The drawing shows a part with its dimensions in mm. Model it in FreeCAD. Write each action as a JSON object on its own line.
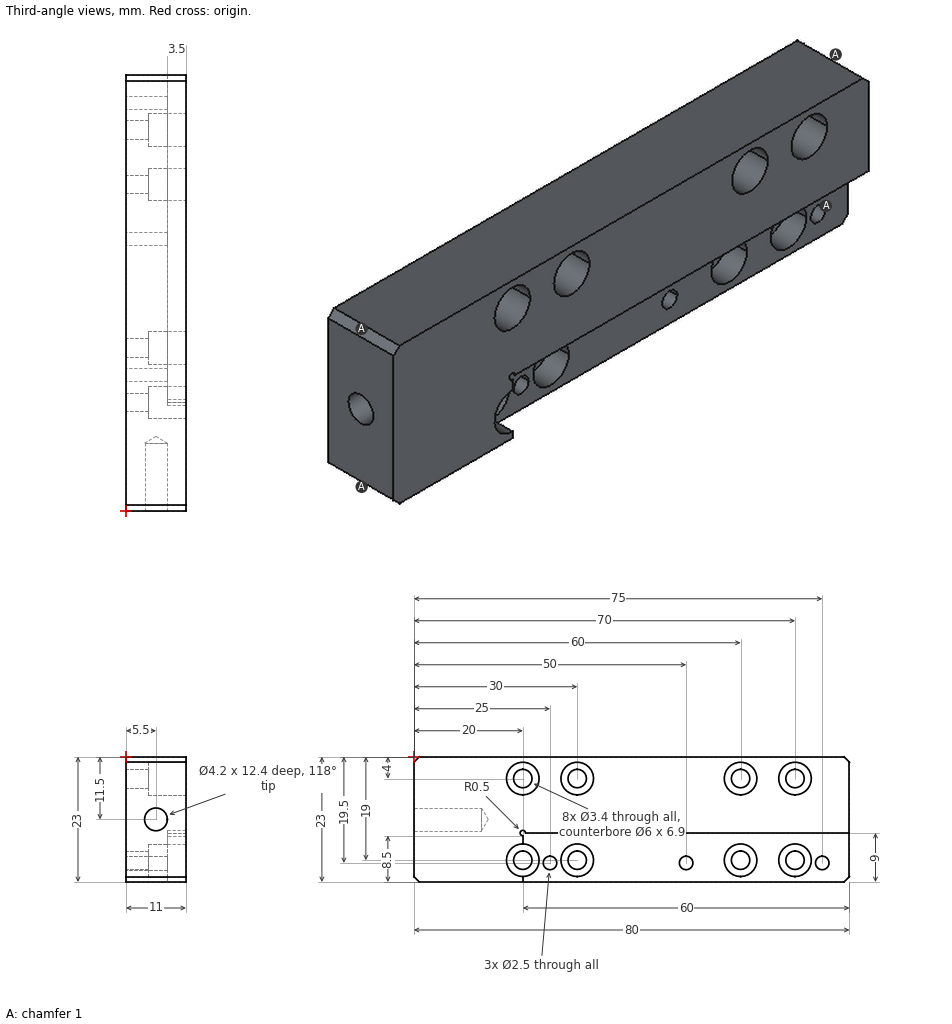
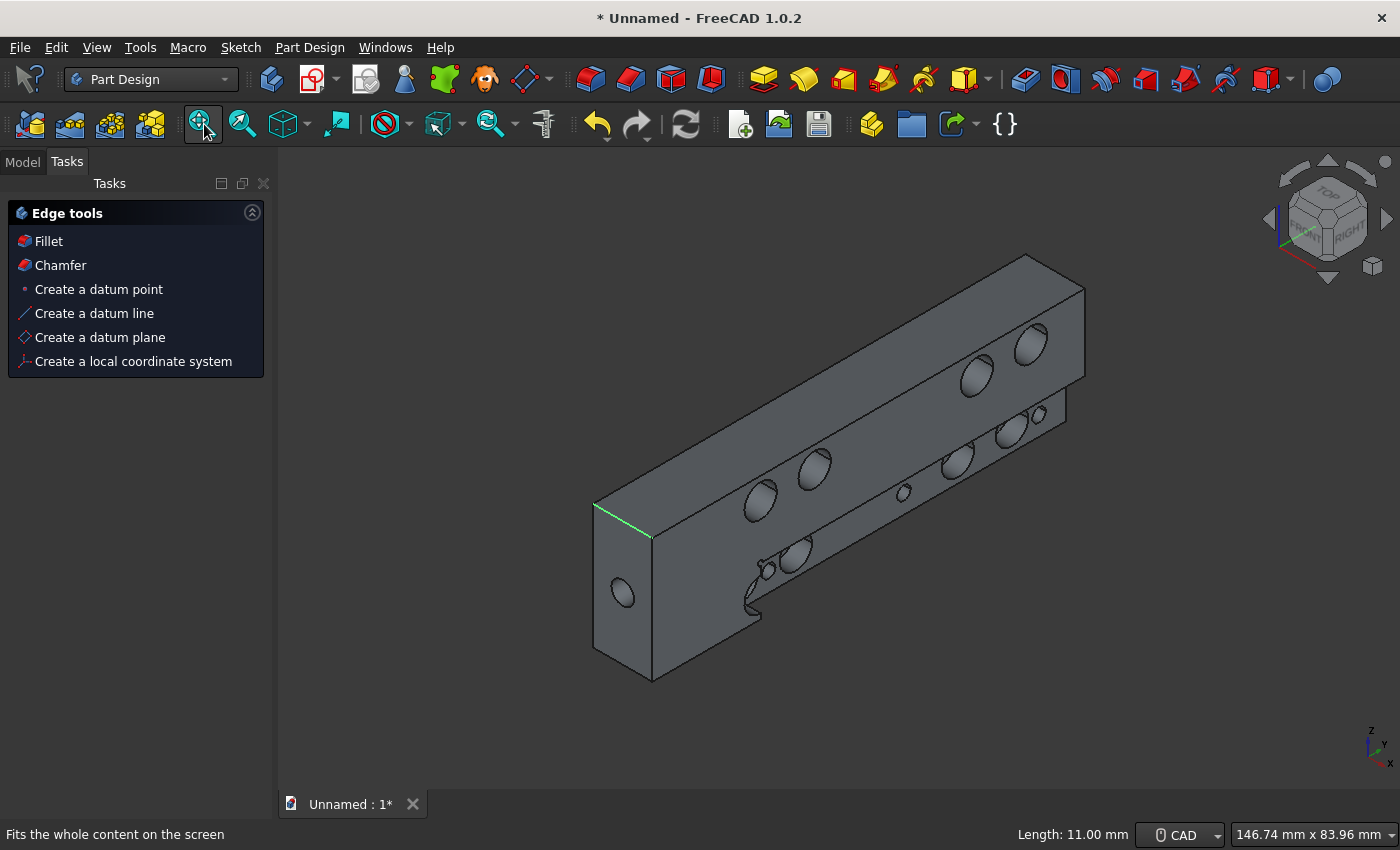
{"action": "key", "text": "1"}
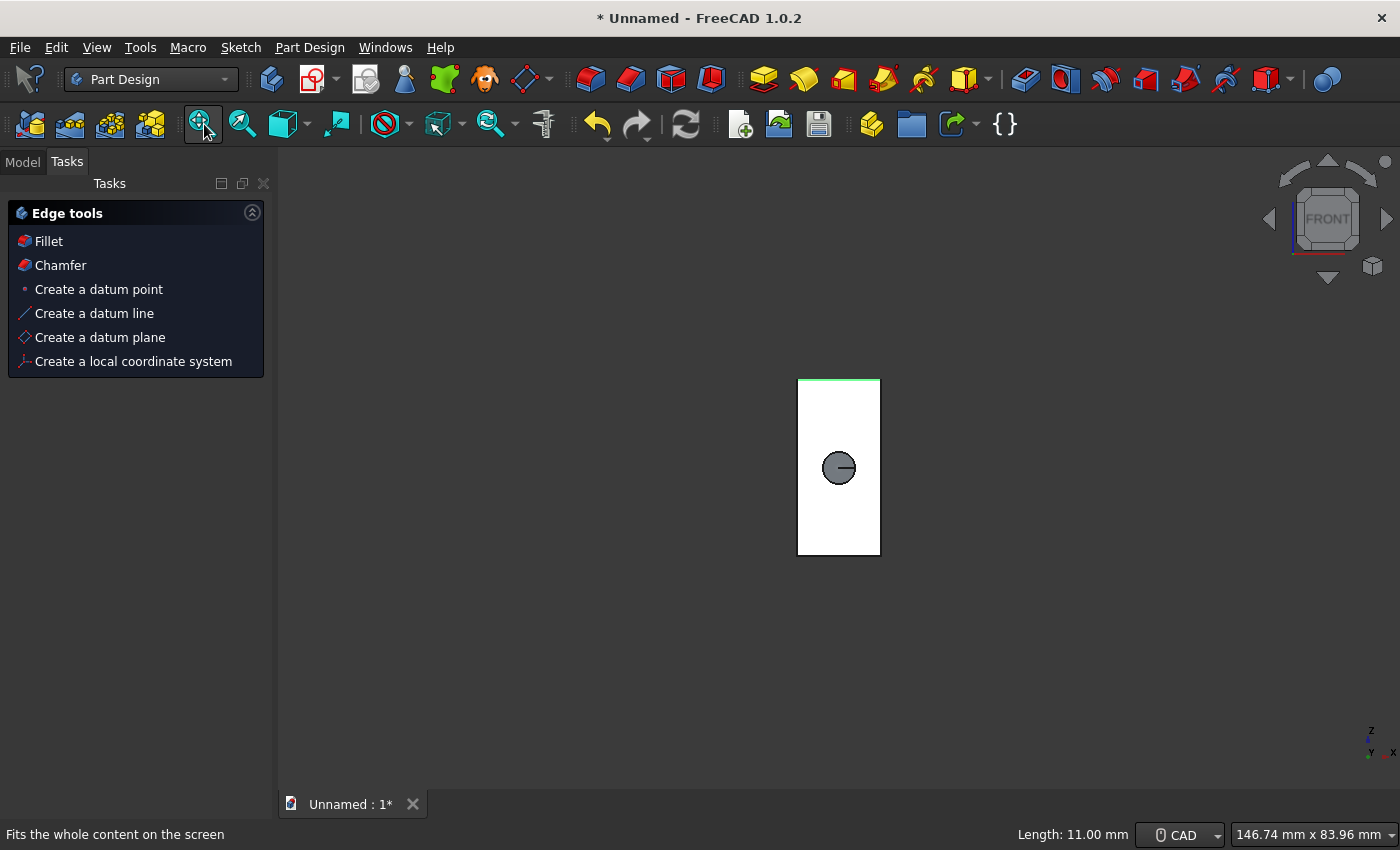
{"action": "left_click", "coordinate": [204, 124]}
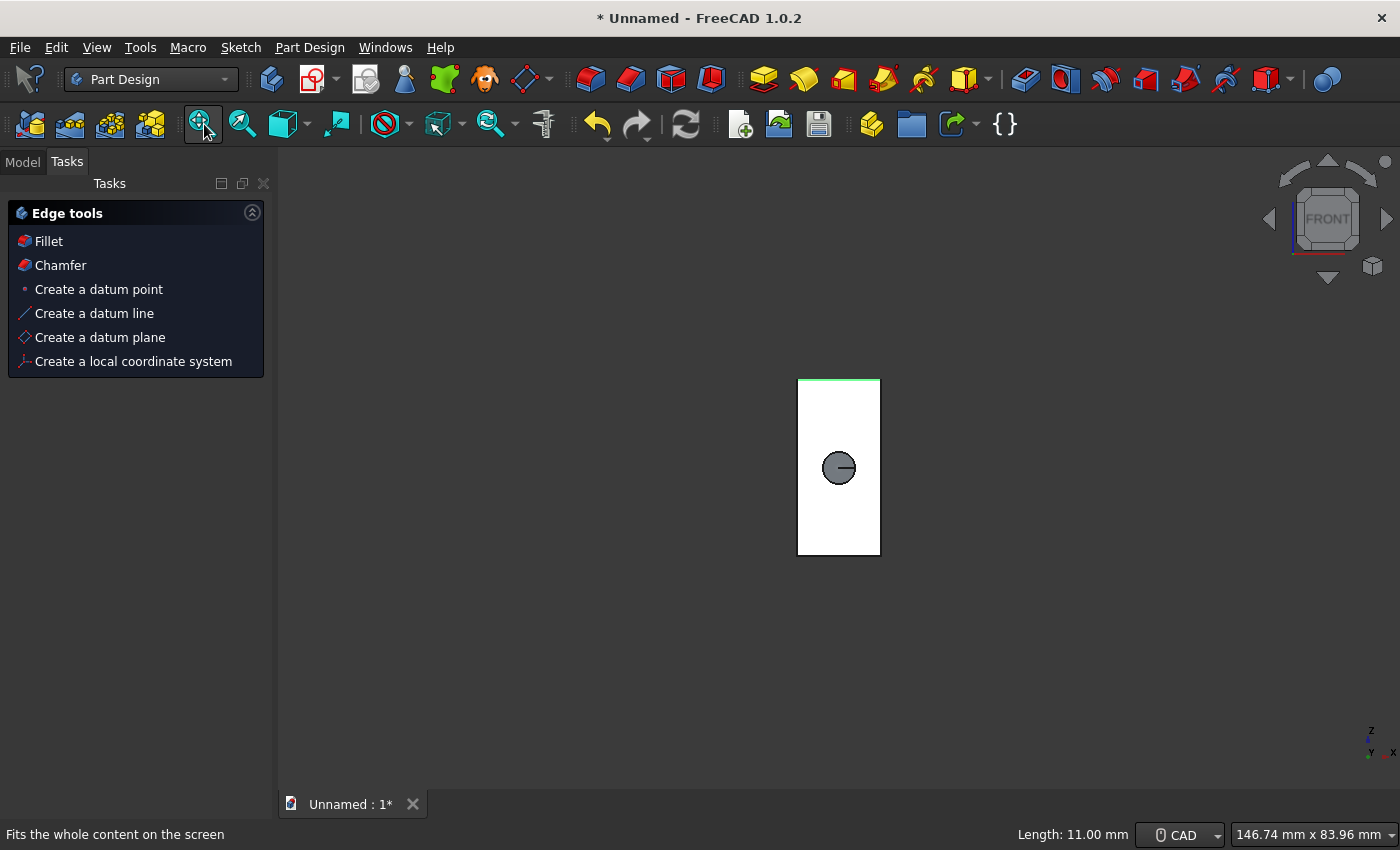
{"action": "key", "text": "3"}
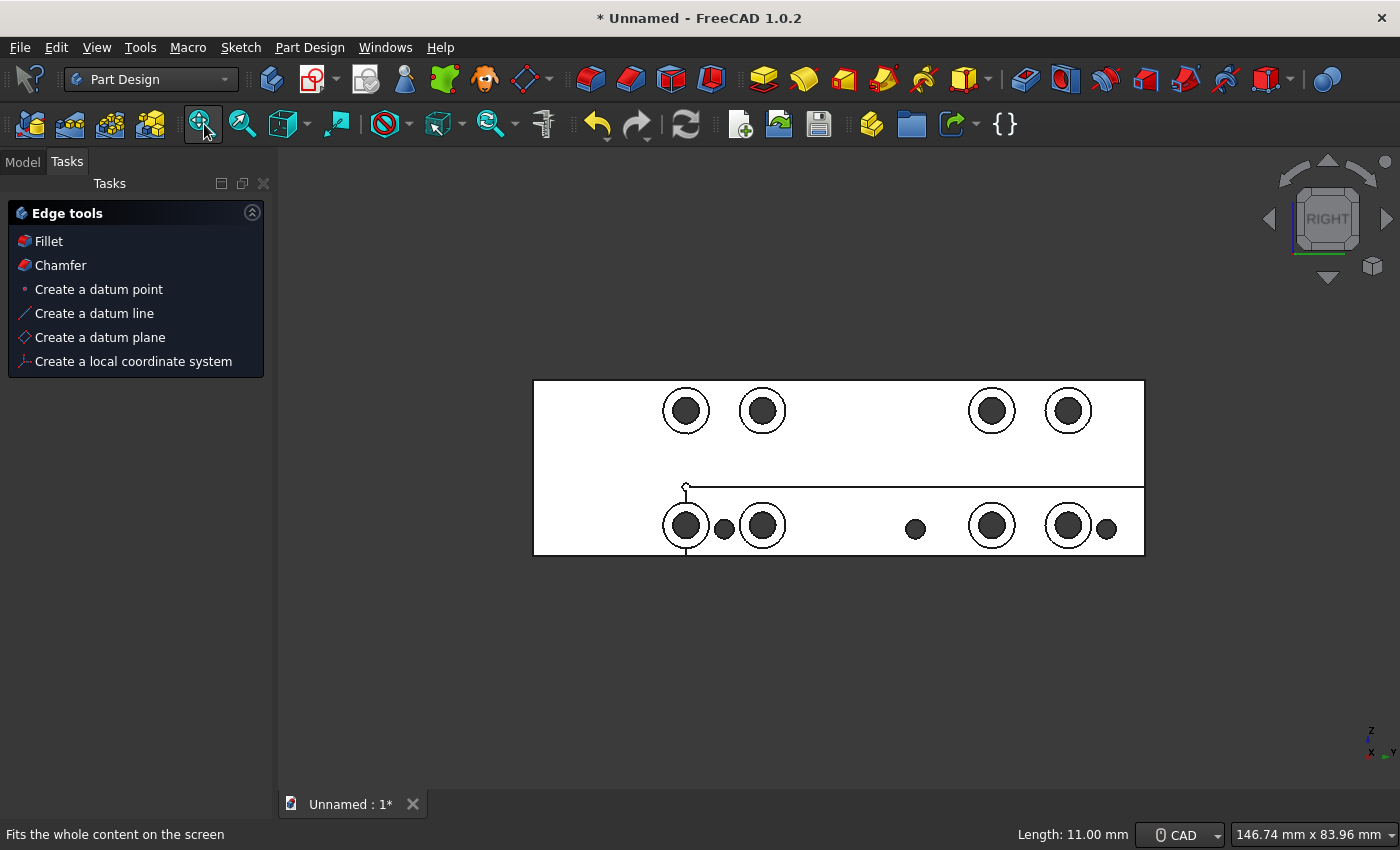
{"action": "key", "text": "5"}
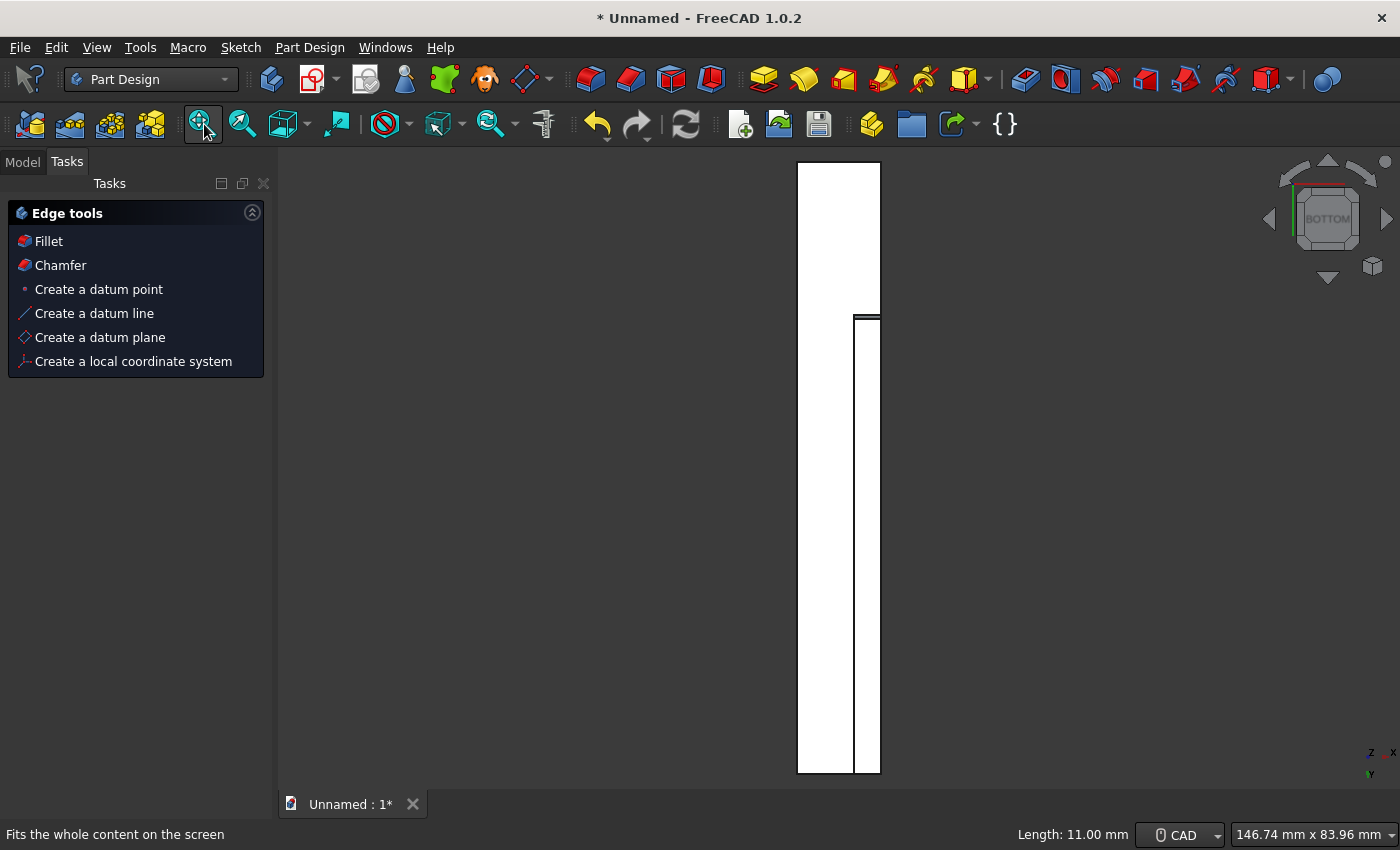
{"action": "key", "text": "4"}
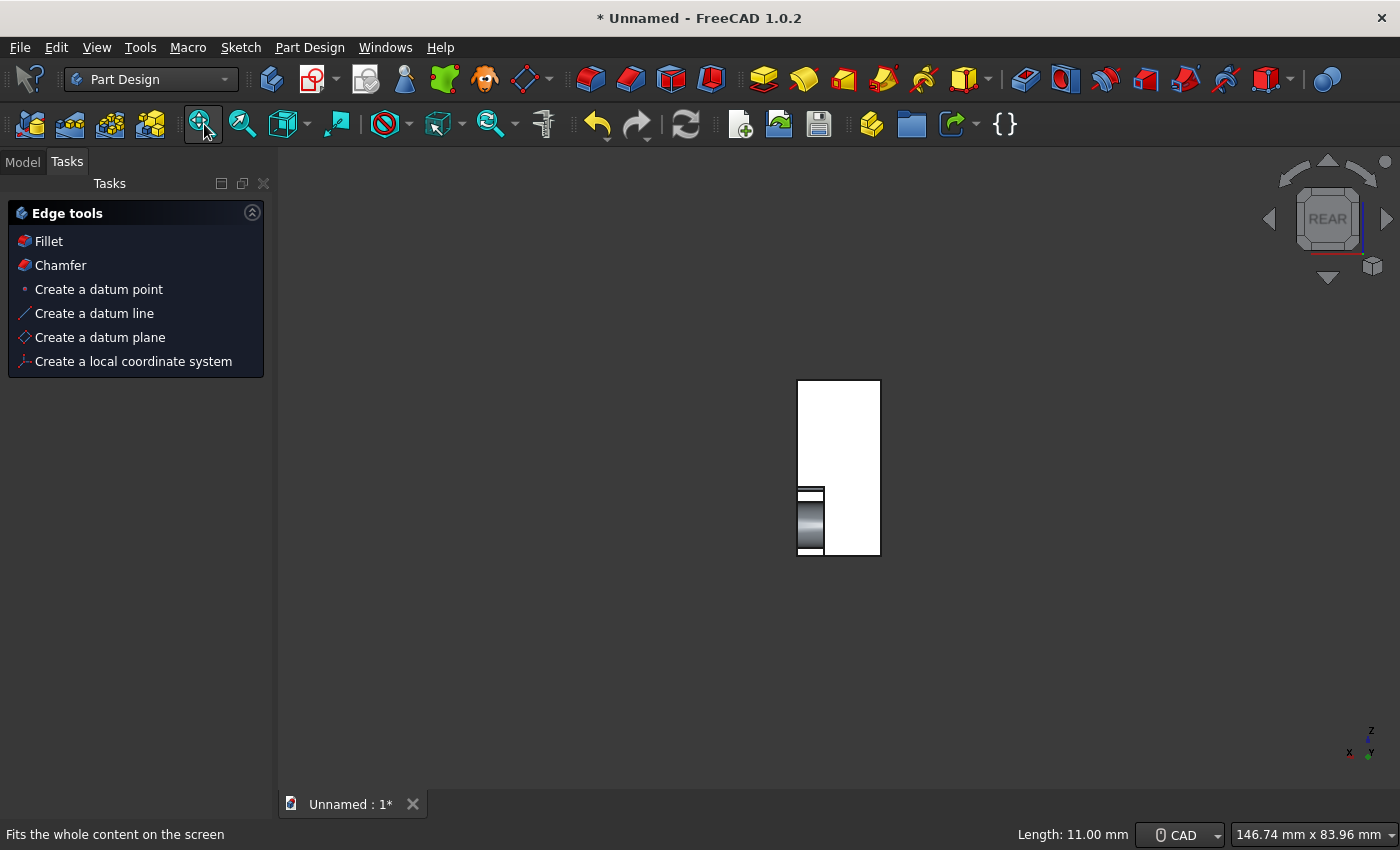
{"action": "left_click", "coordinate": [204, 124]}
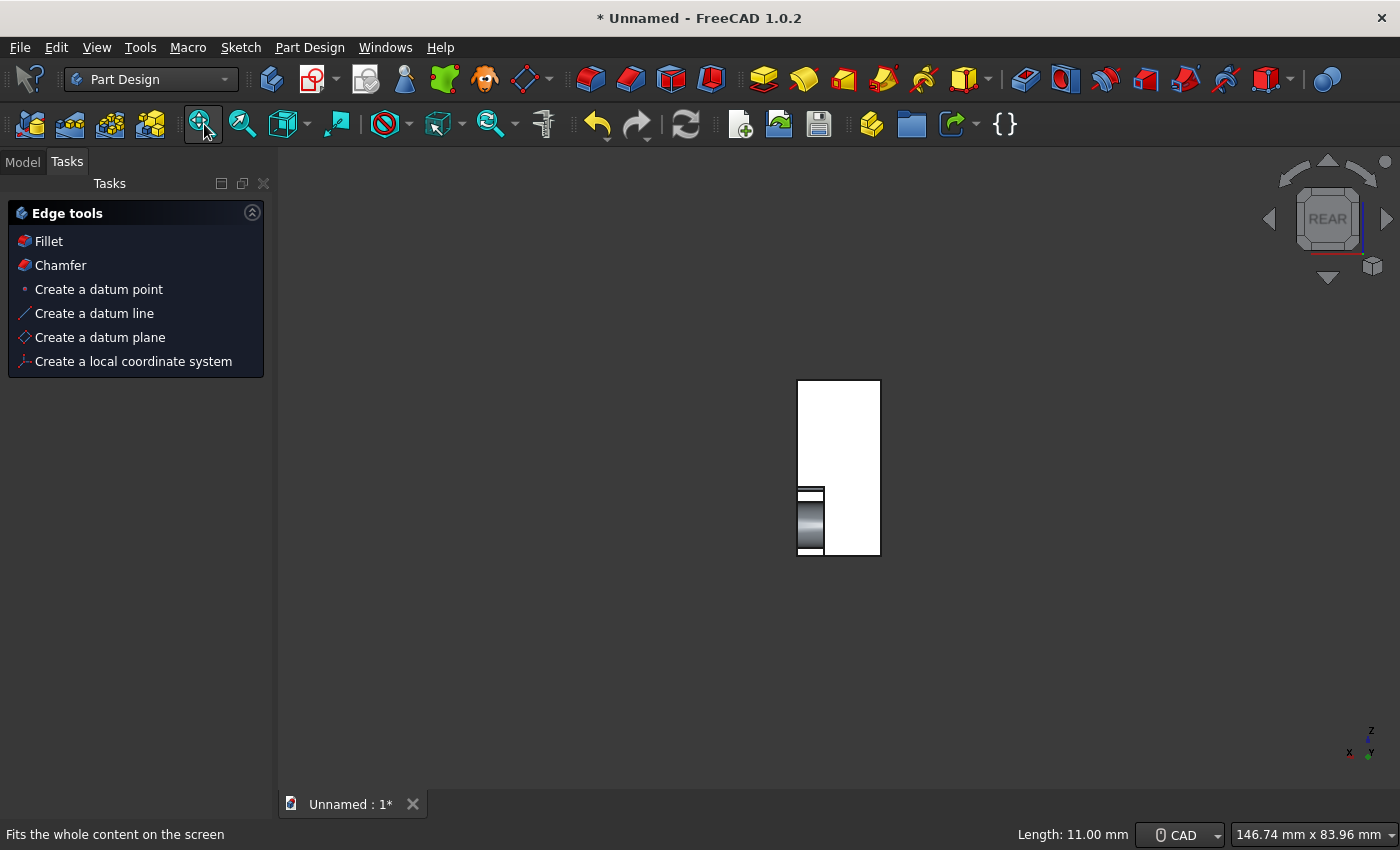
{"action": "left_click", "coordinate": [852, 555], "text": "ctrl"}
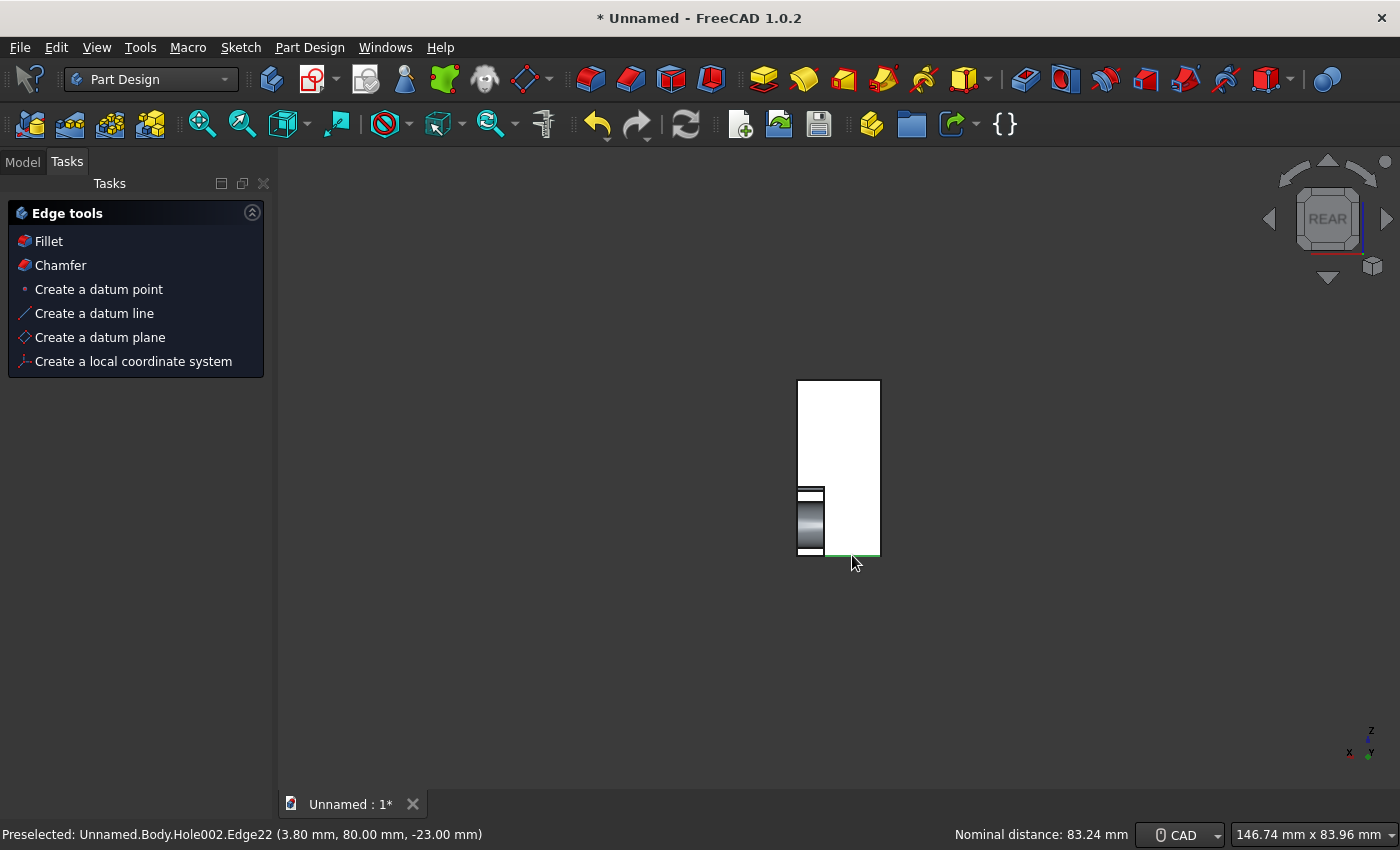
{"action": "key", "text": "6"}